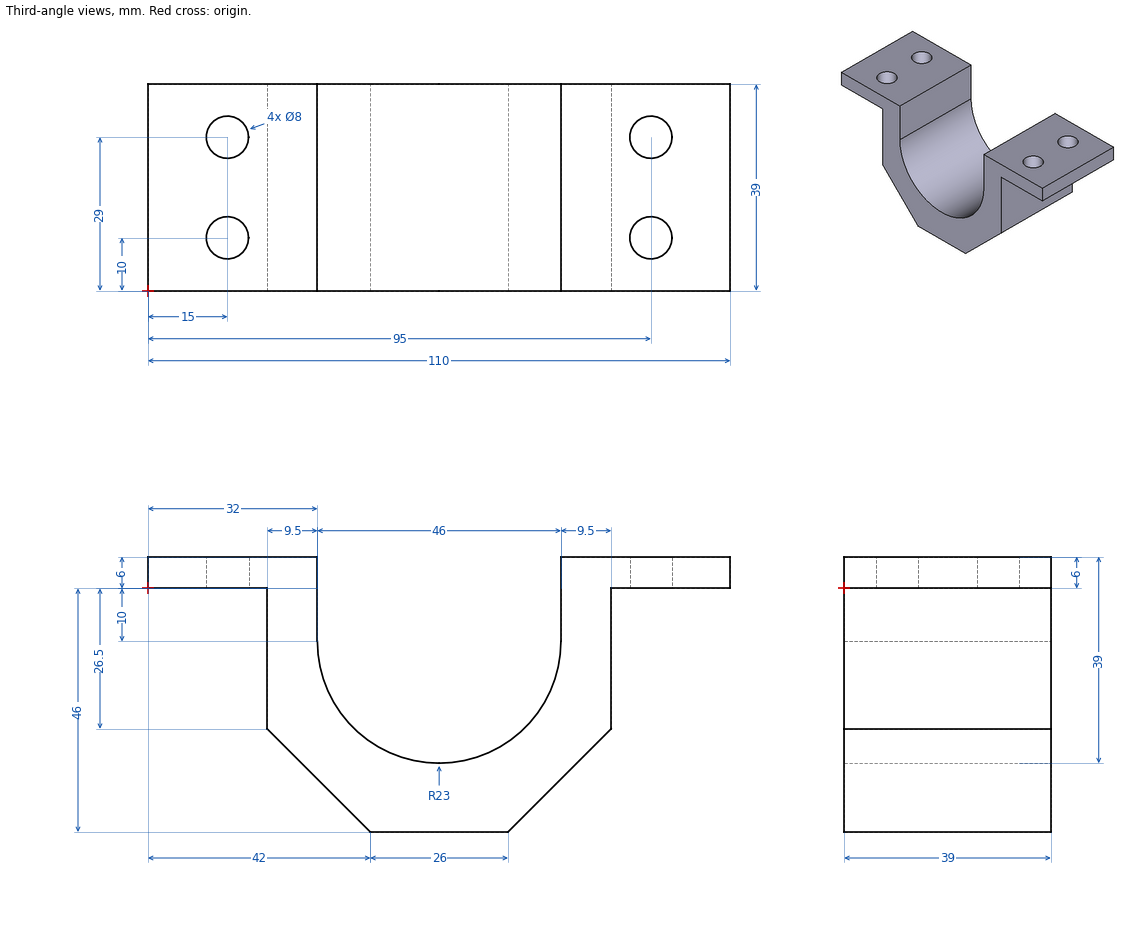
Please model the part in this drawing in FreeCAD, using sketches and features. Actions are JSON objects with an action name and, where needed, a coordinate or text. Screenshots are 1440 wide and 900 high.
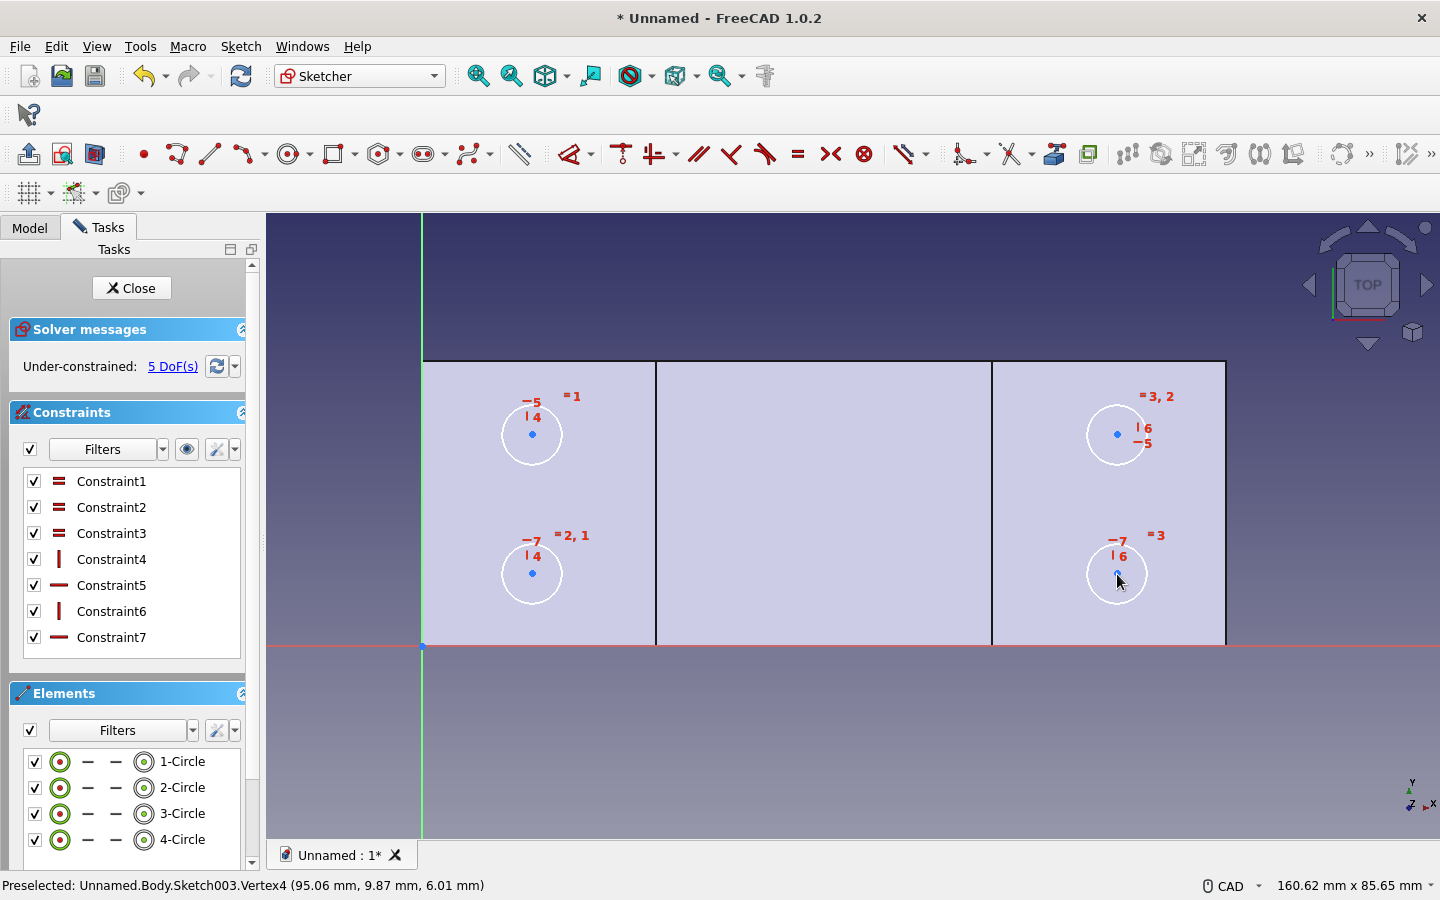
{"action": "key", "text": "d"}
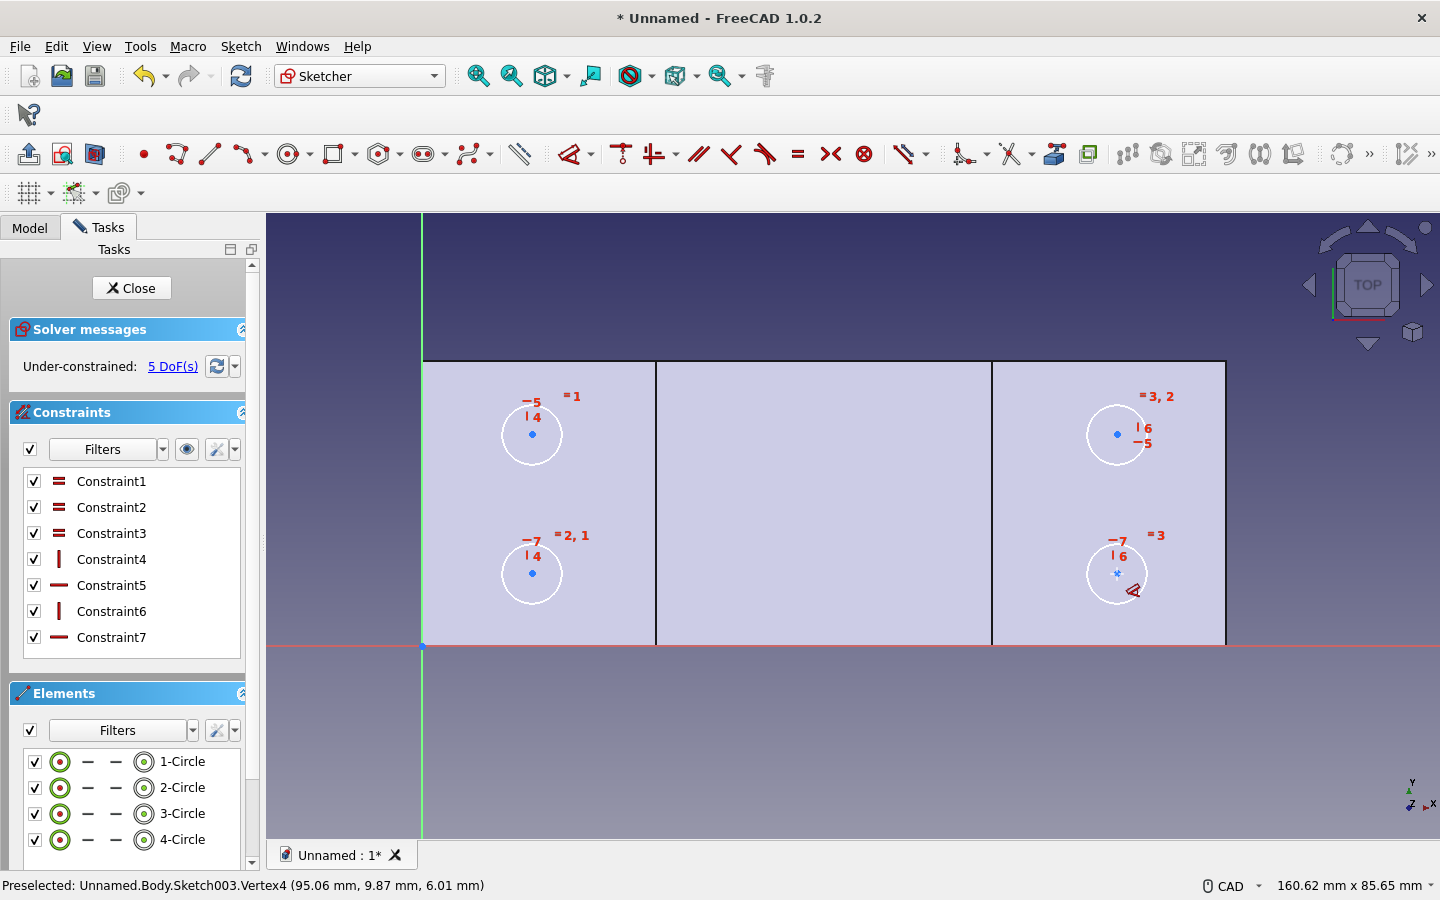
{"action": "left_click", "coordinate": [553, 414]}
{"action": "left_click", "coordinate": [576, 391]}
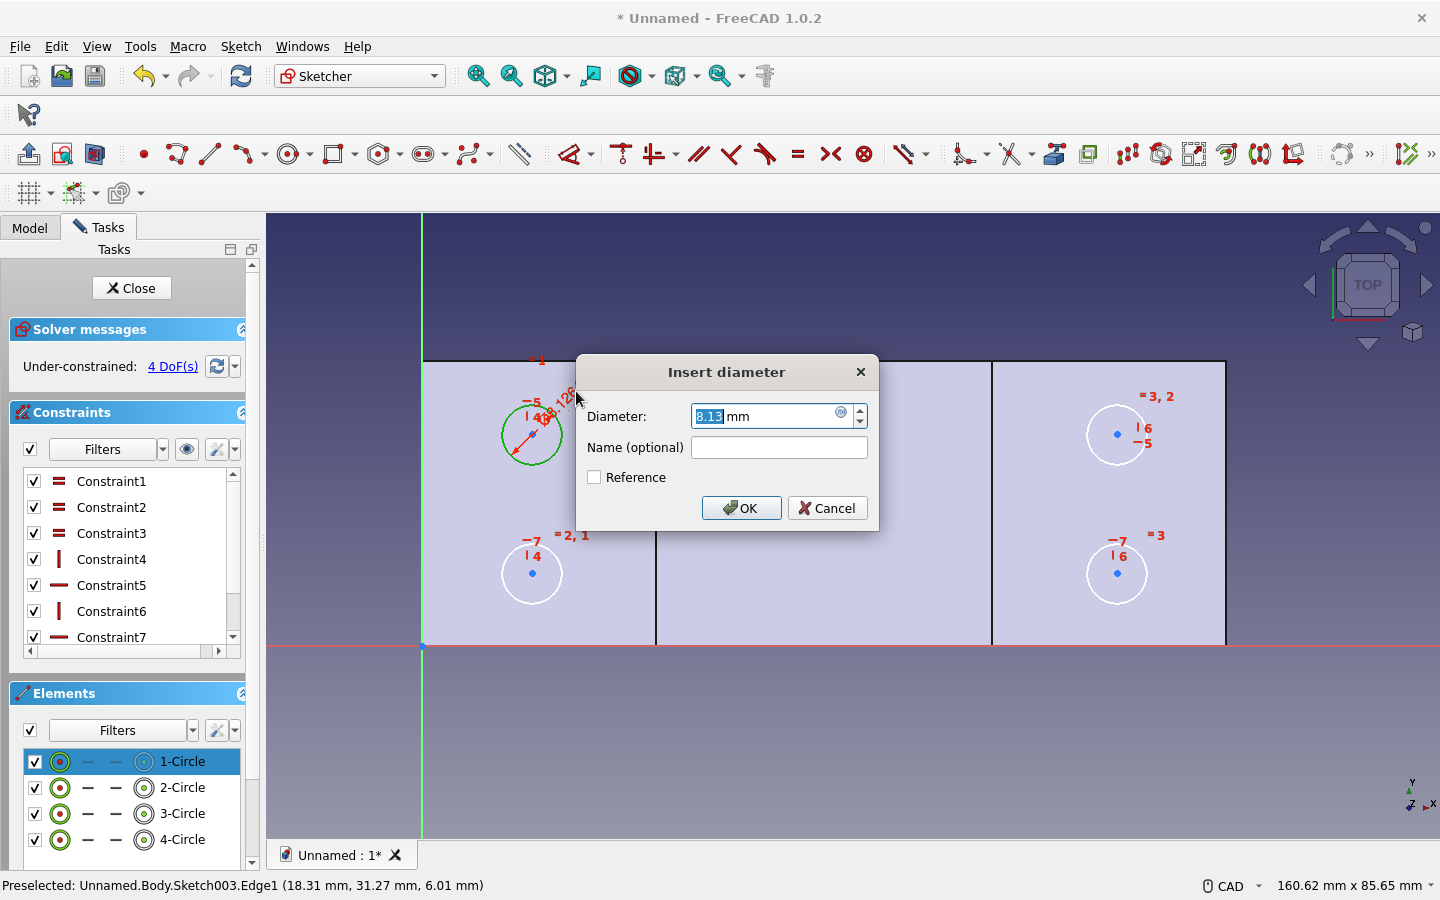
{"action": "type", "text": "8"}
{"action": "key", "text": "Return"}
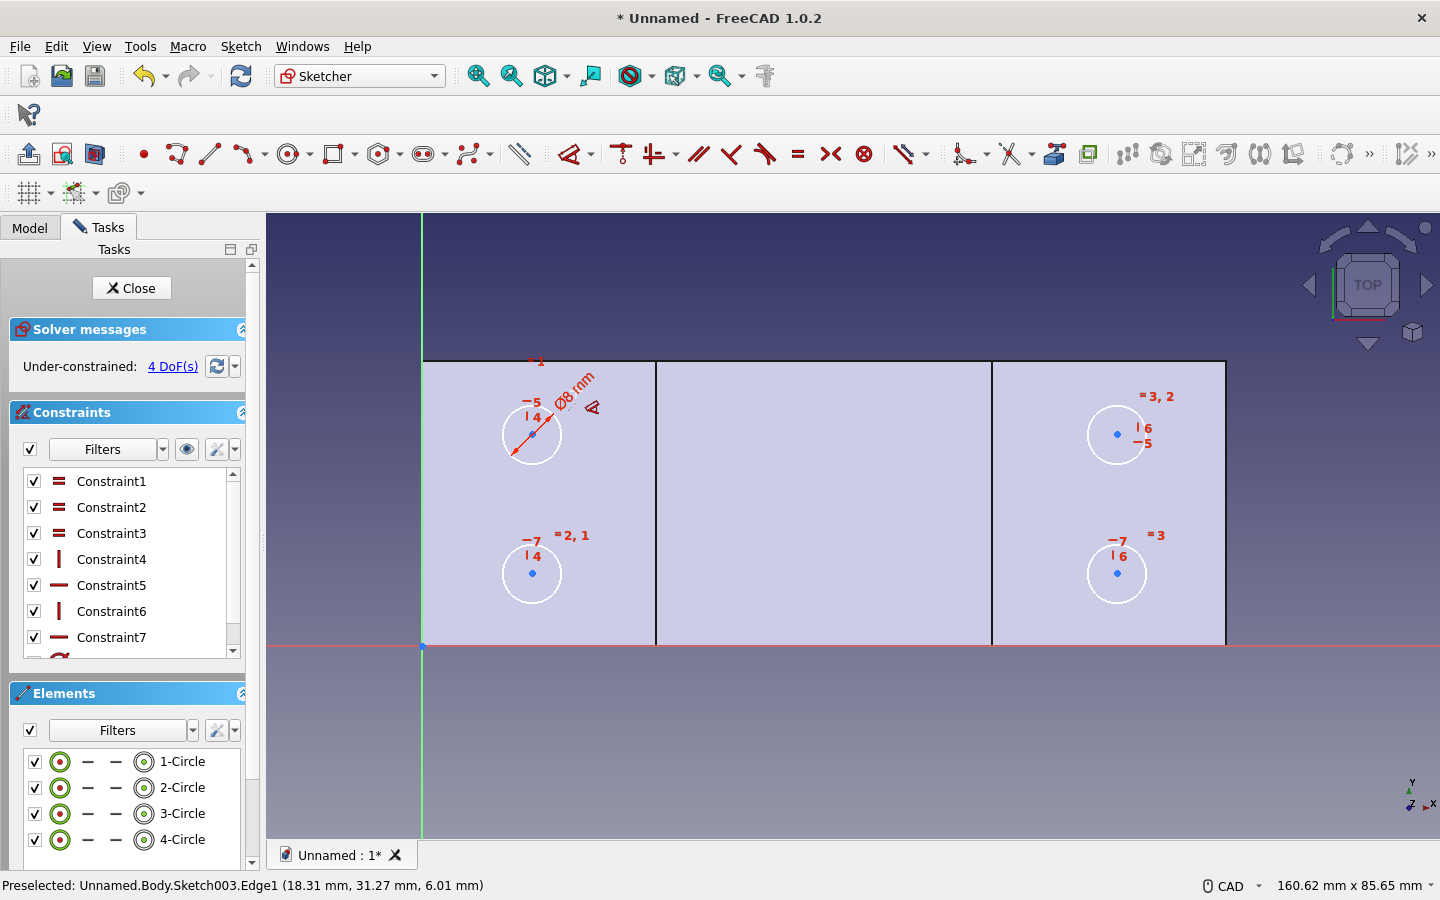
{"action": "left_click", "coordinate": [532, 435]}
{"action": "left_click", "coordinate": [477, 680]}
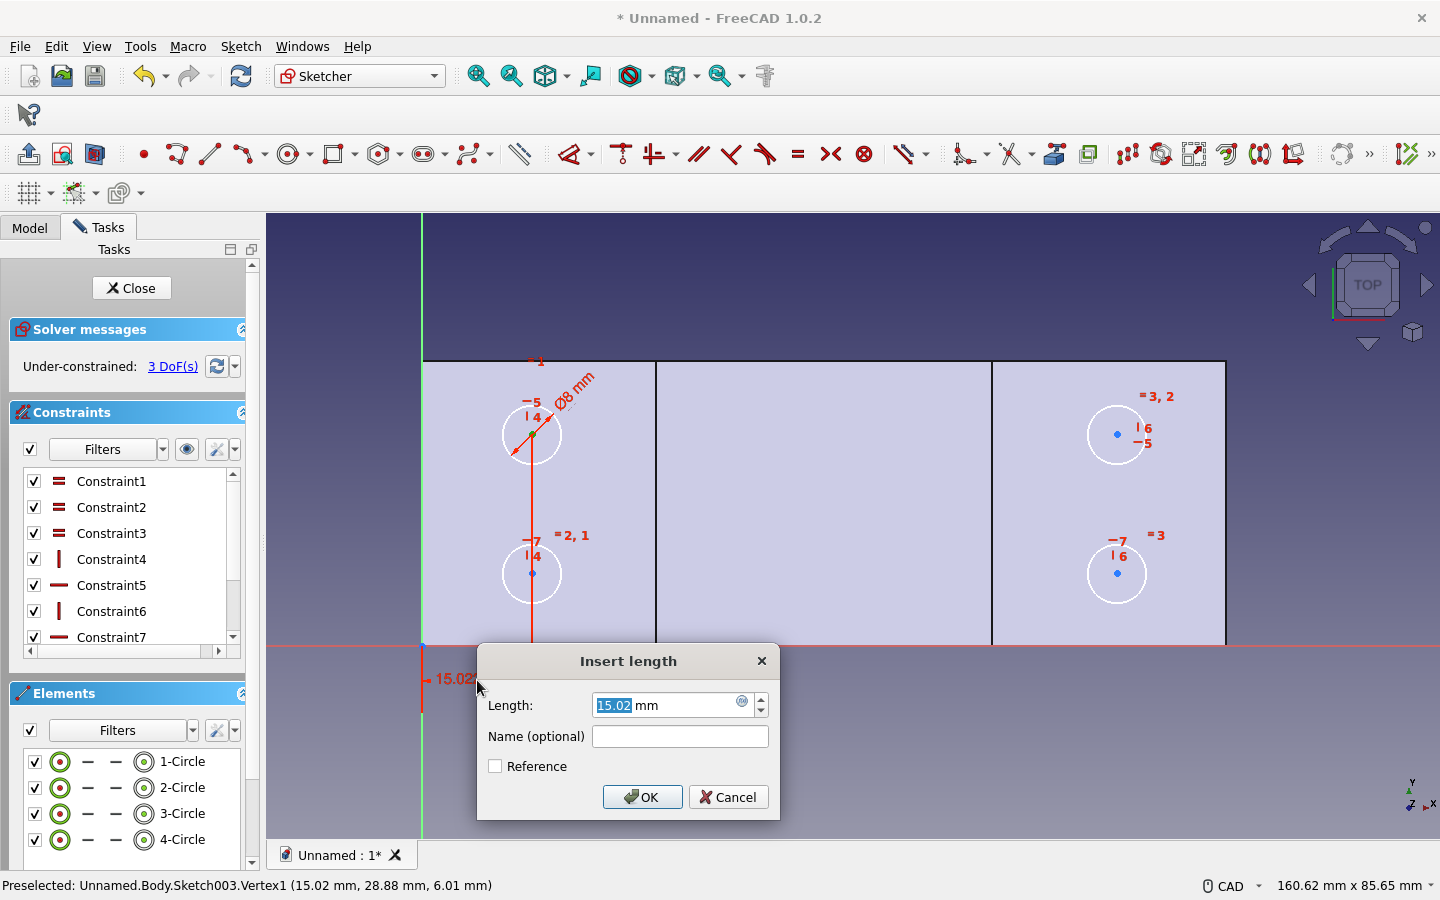
{"action": "type", "text": "15"}
{"action": "key", "text": "Return"}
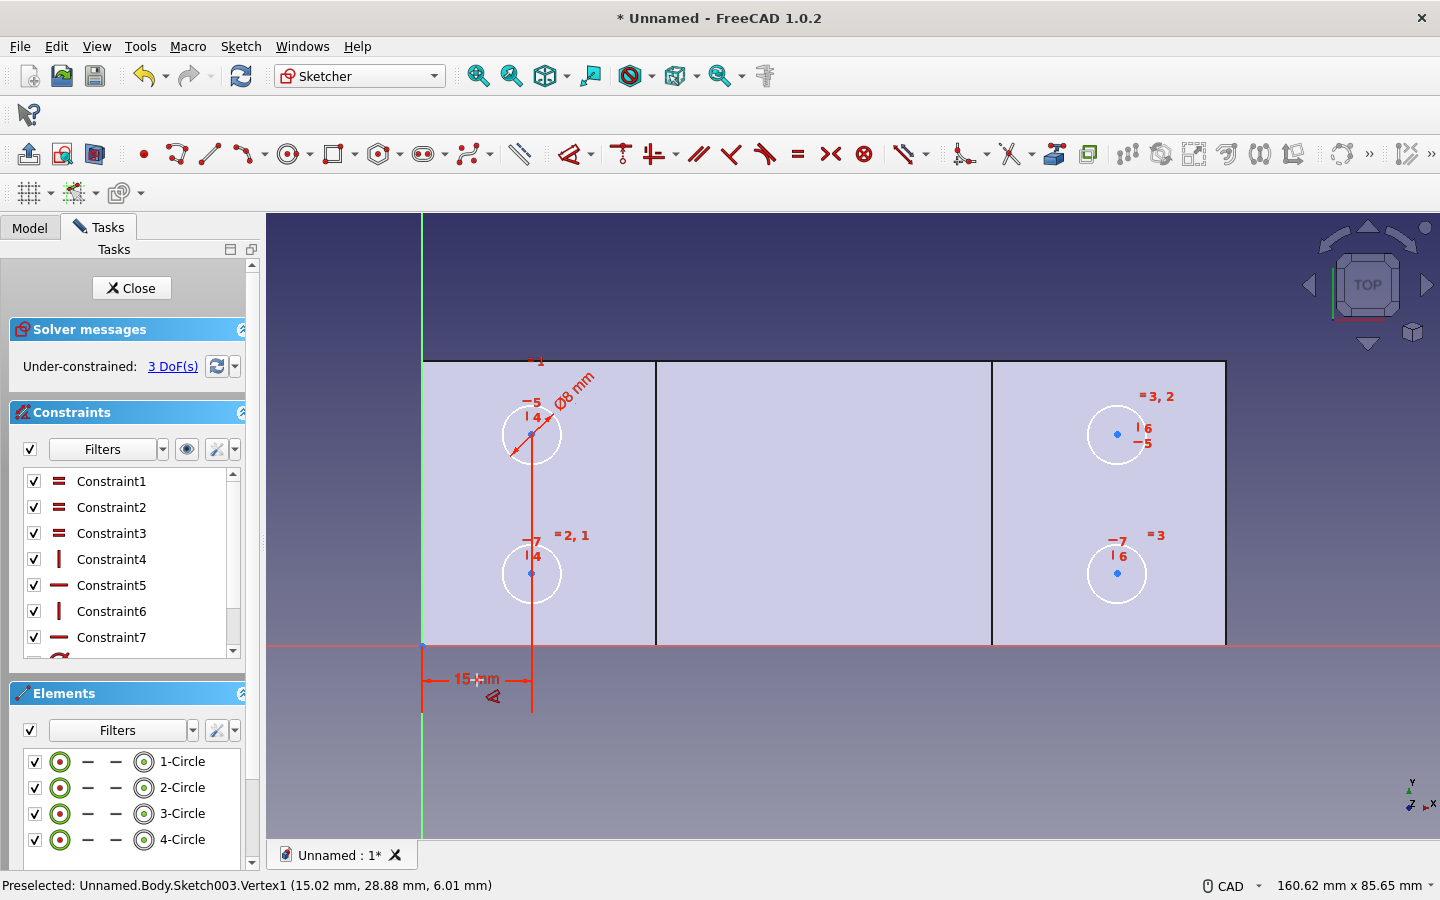
{"action": "left_click", "coordinate": [532, 435]}
{"action": "left_click", "coordinate": [388, 541]}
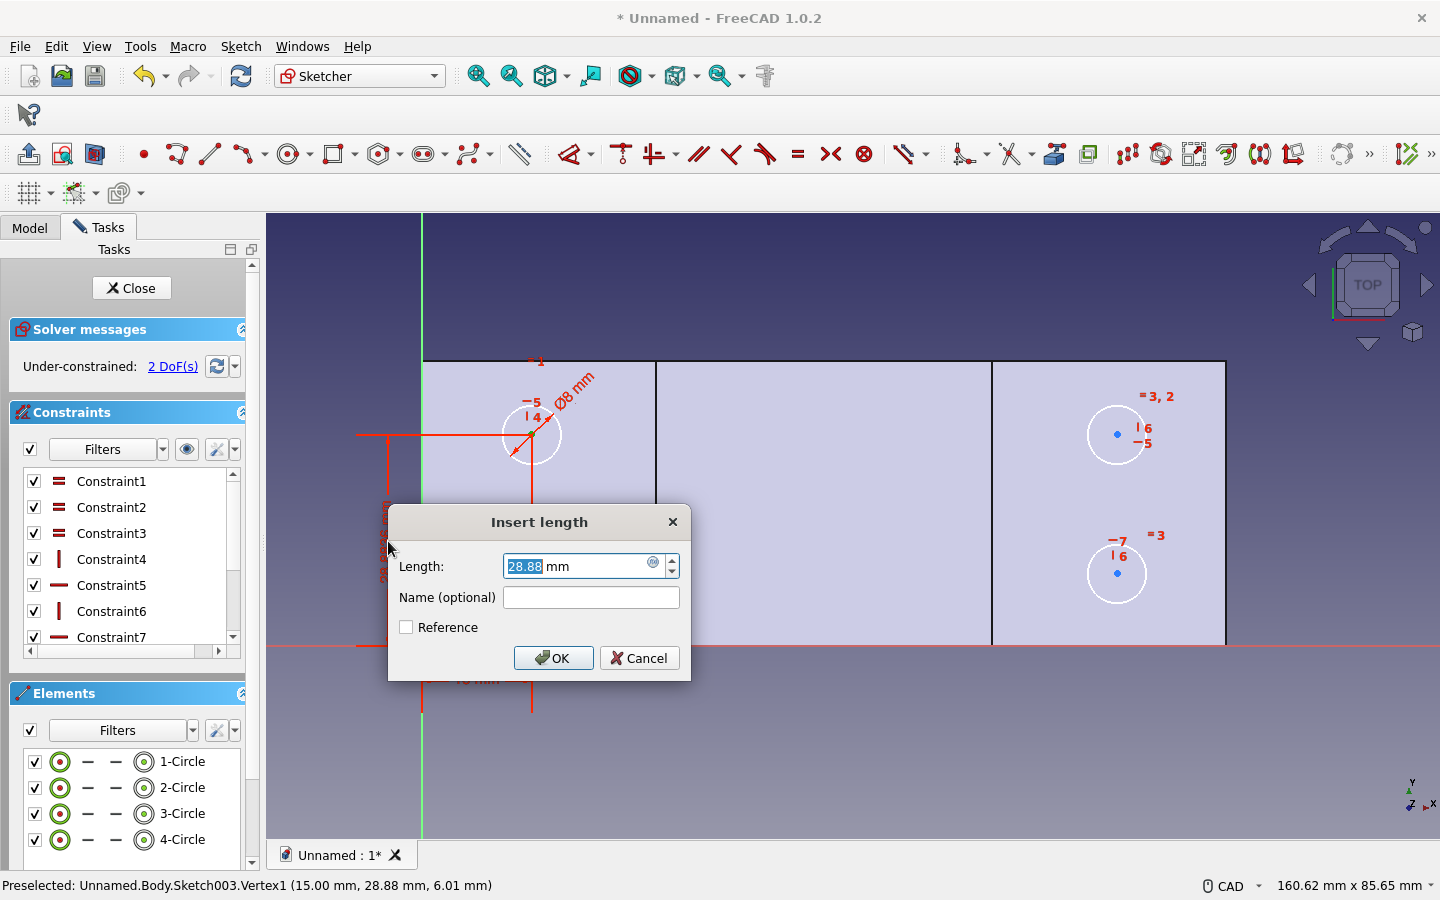
{"action": "type", "text": "29"}
{"action": "key", "text": "Return"}